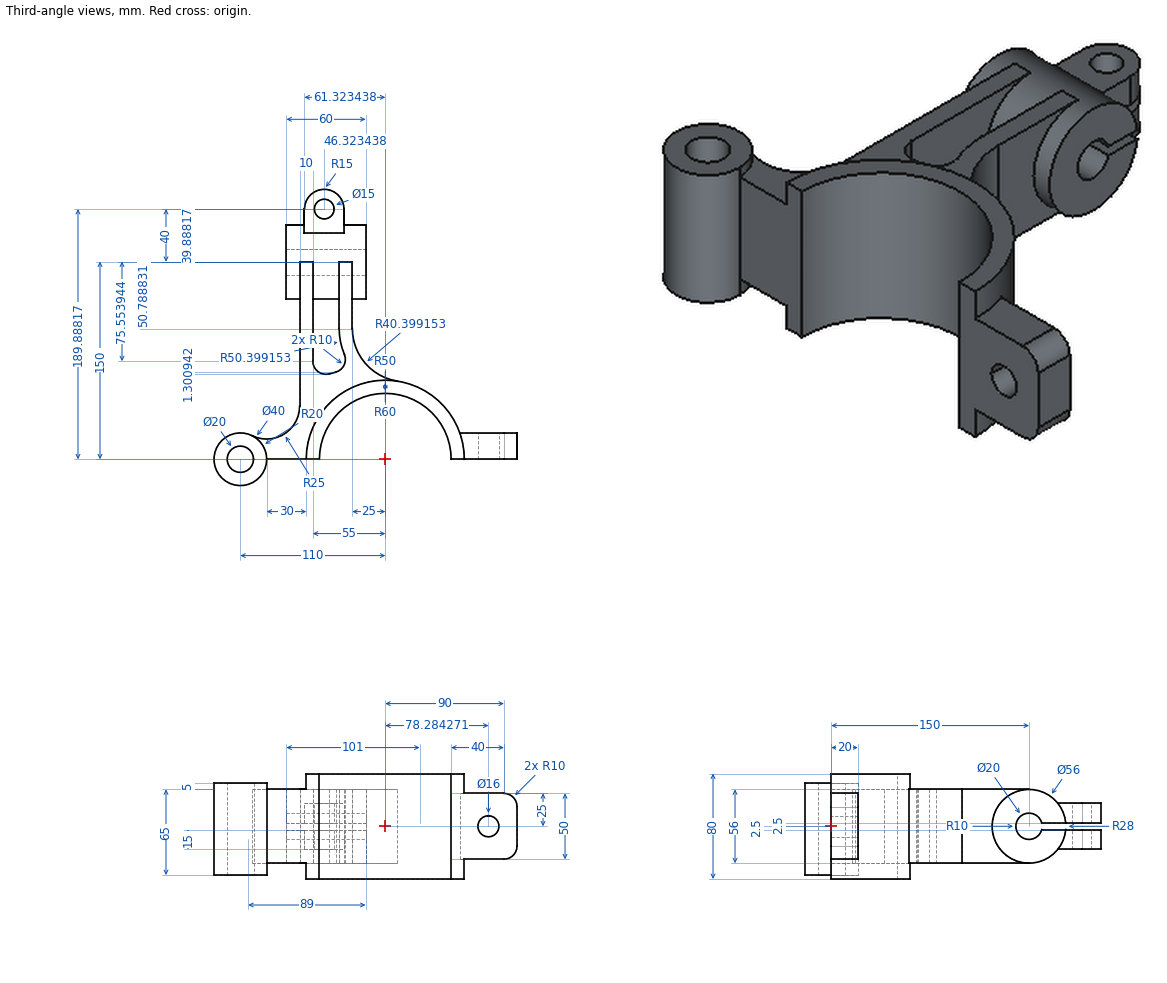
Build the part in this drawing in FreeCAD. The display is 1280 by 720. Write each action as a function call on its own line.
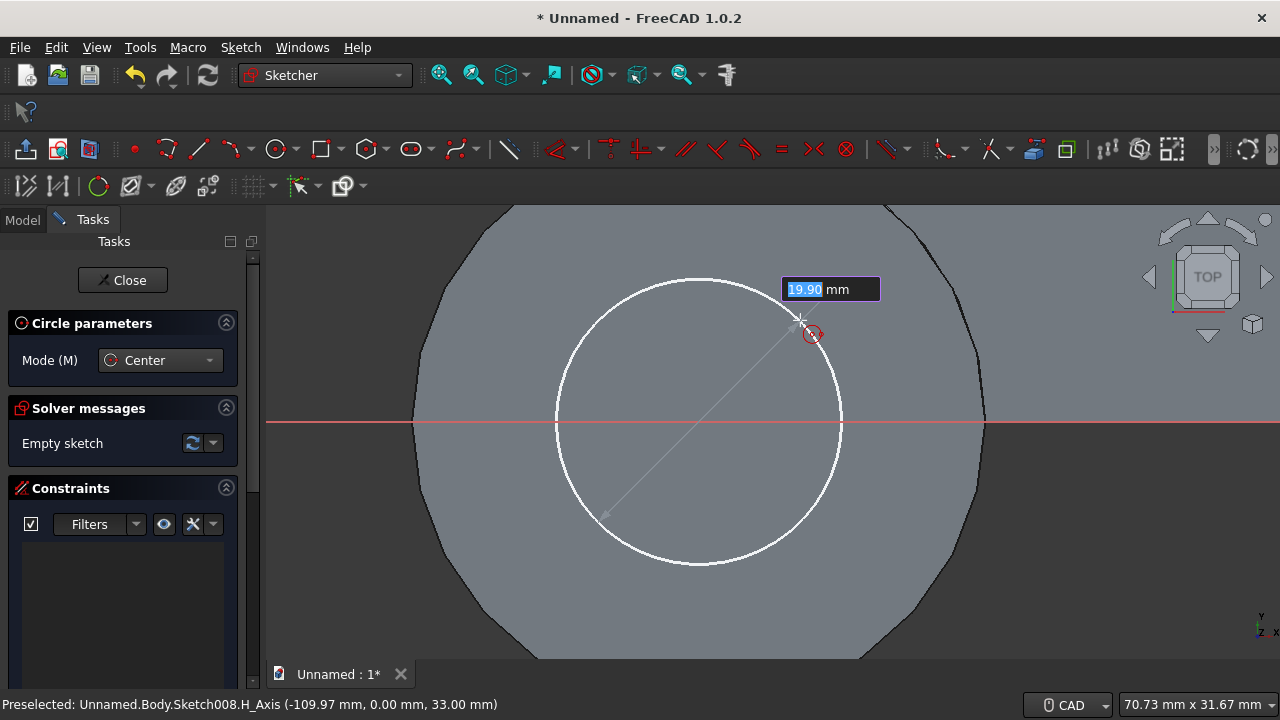
text(20)
key(Return)
key(Escape)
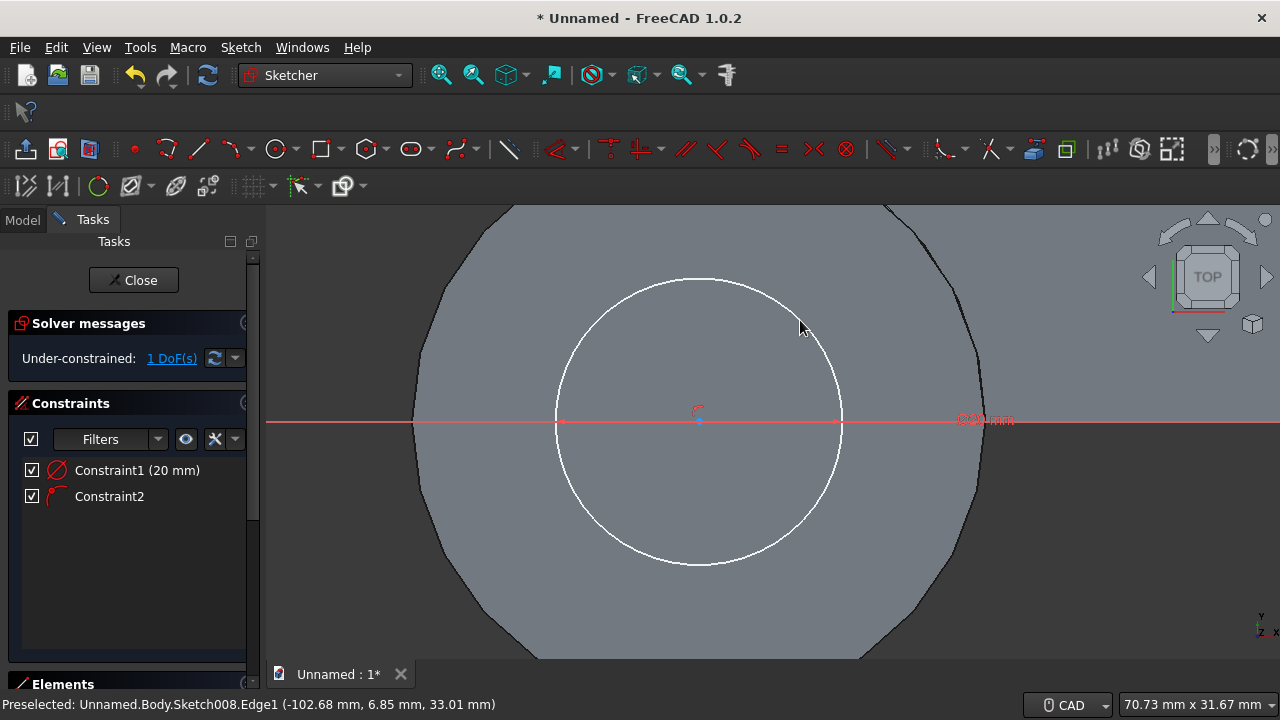
key(d)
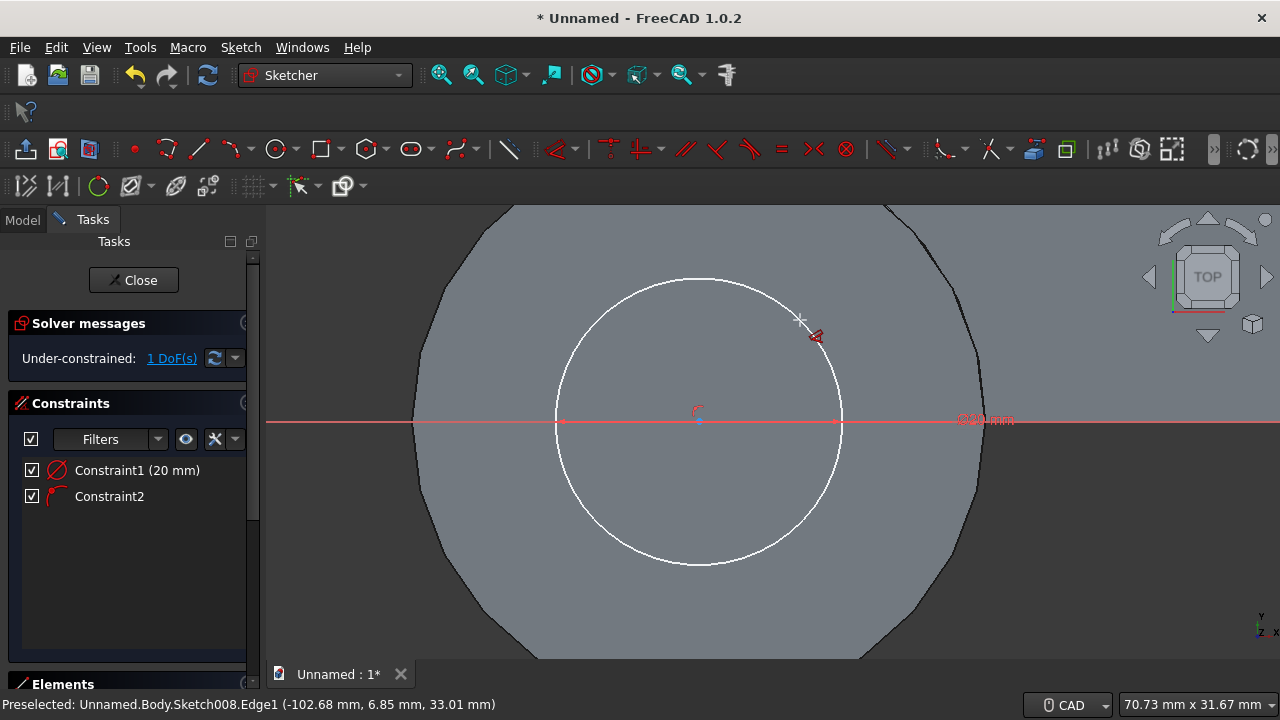
click(699, 422)
click(907, 456)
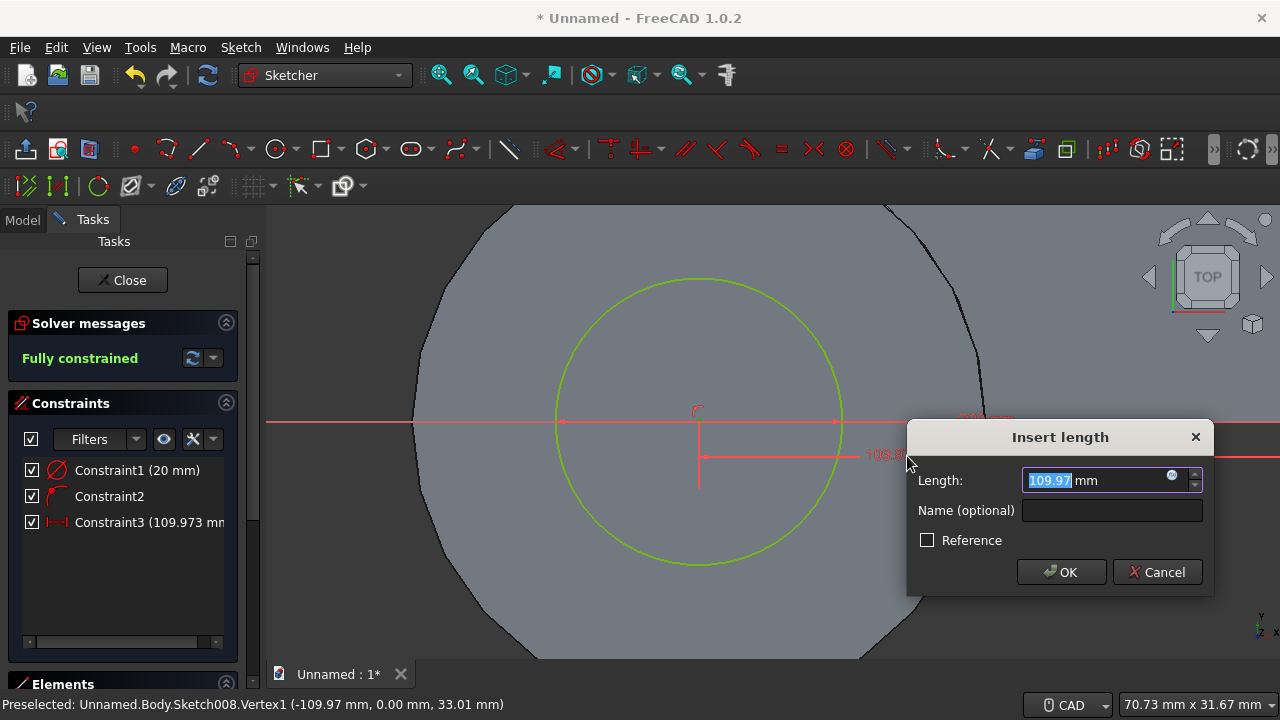
text(110)
key(Return)
key(Escape)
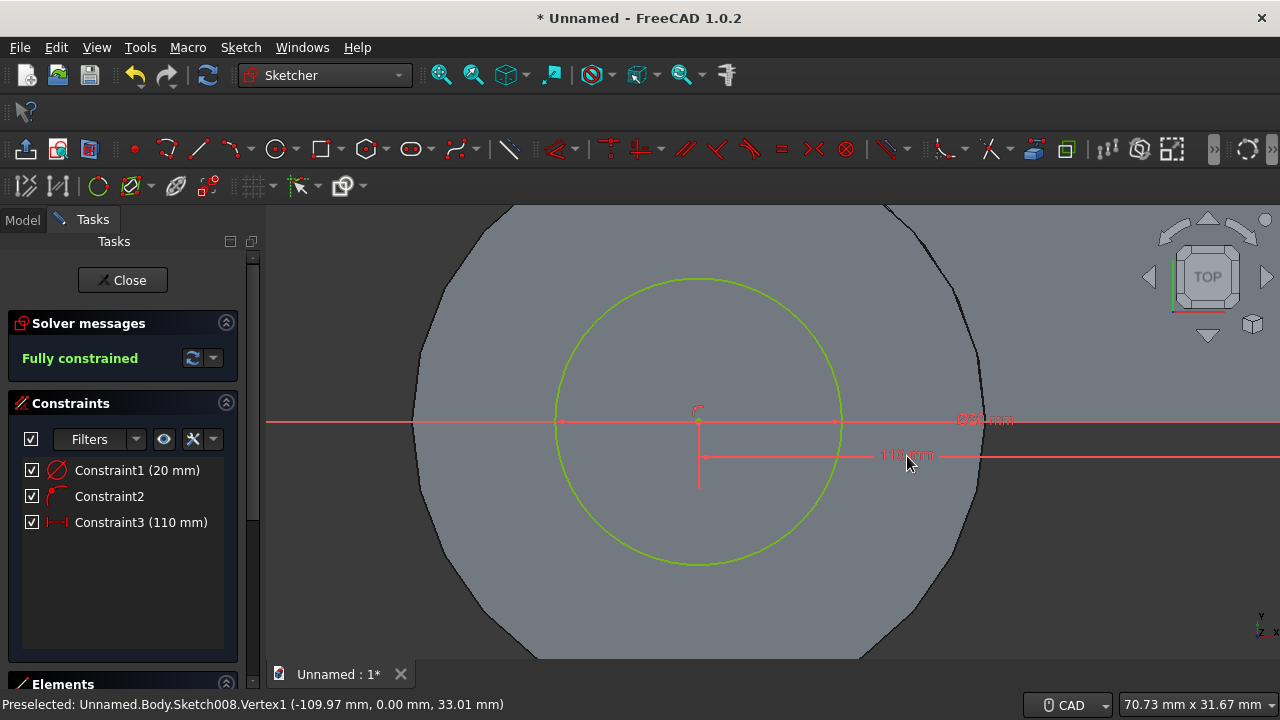
click(123, 280)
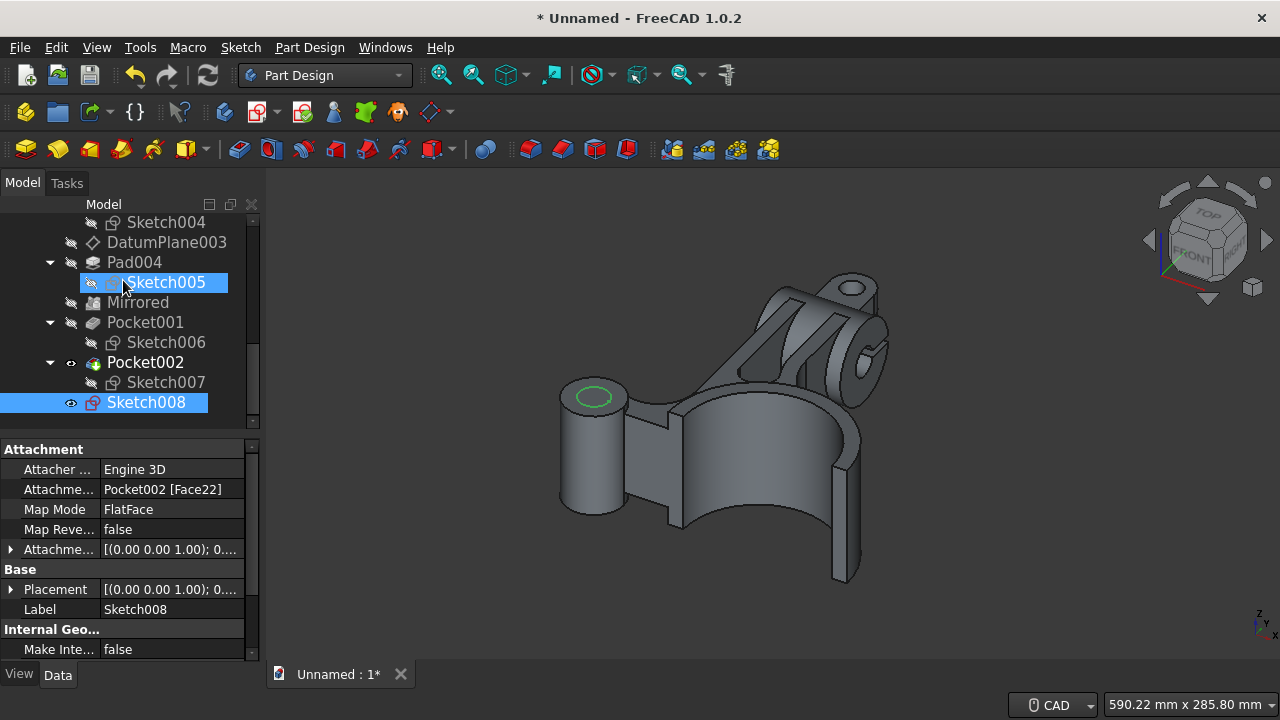
click(240, 150)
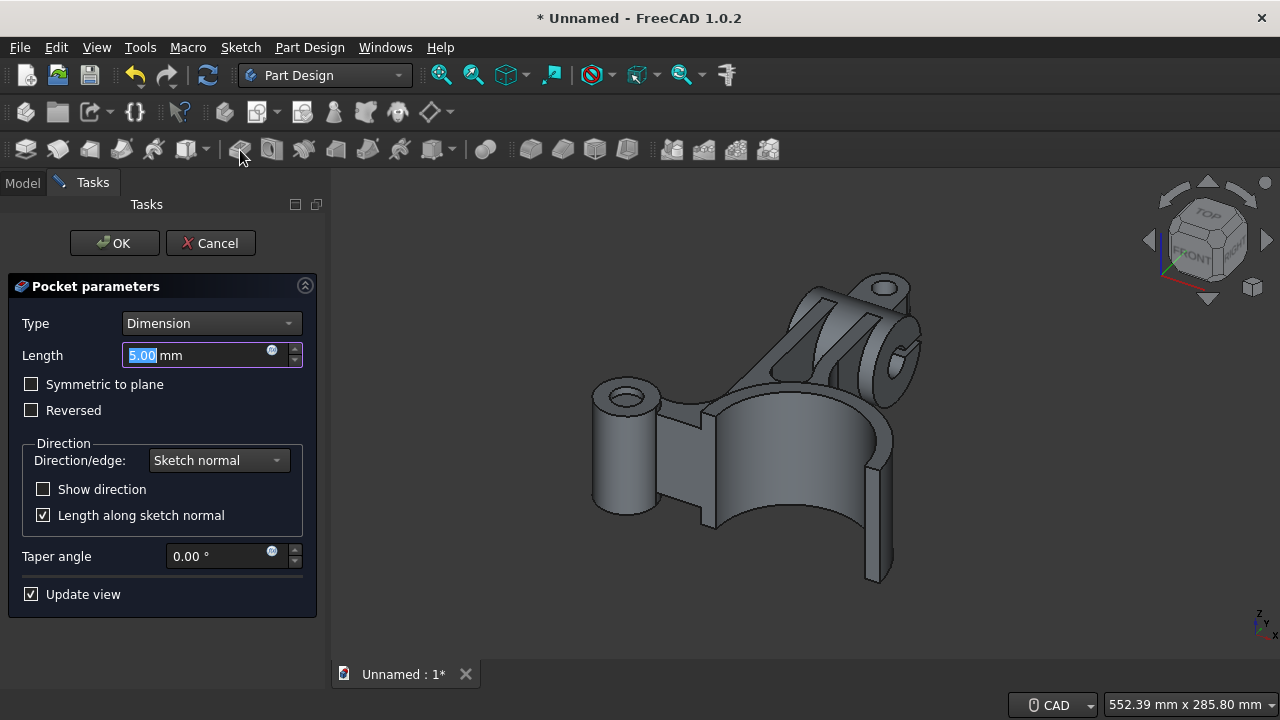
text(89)
key(Tab)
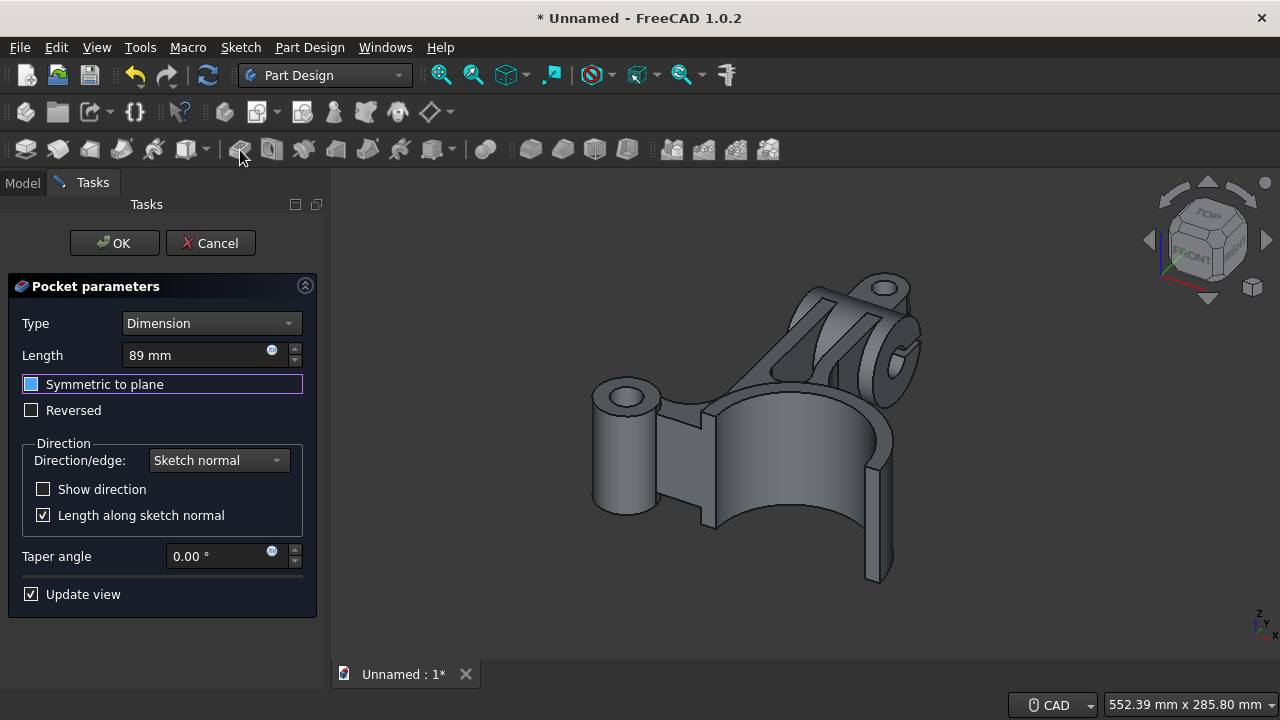
click(115, 243)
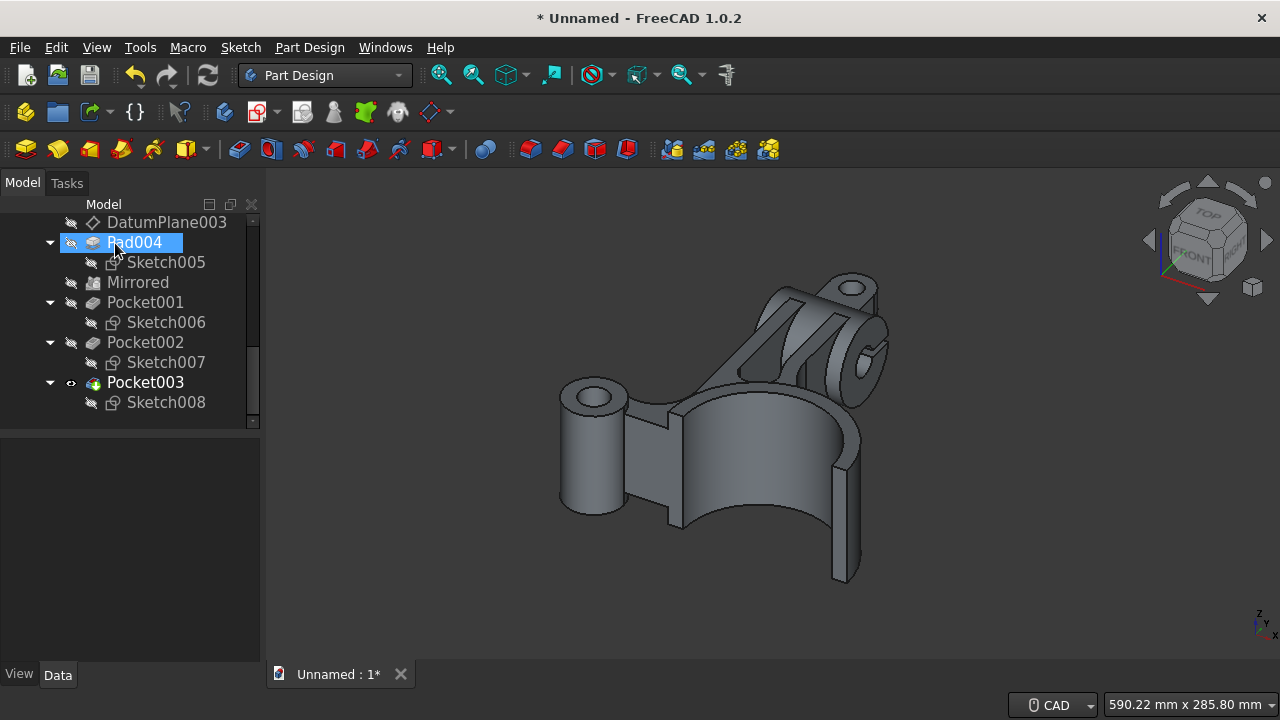
click(258, 112)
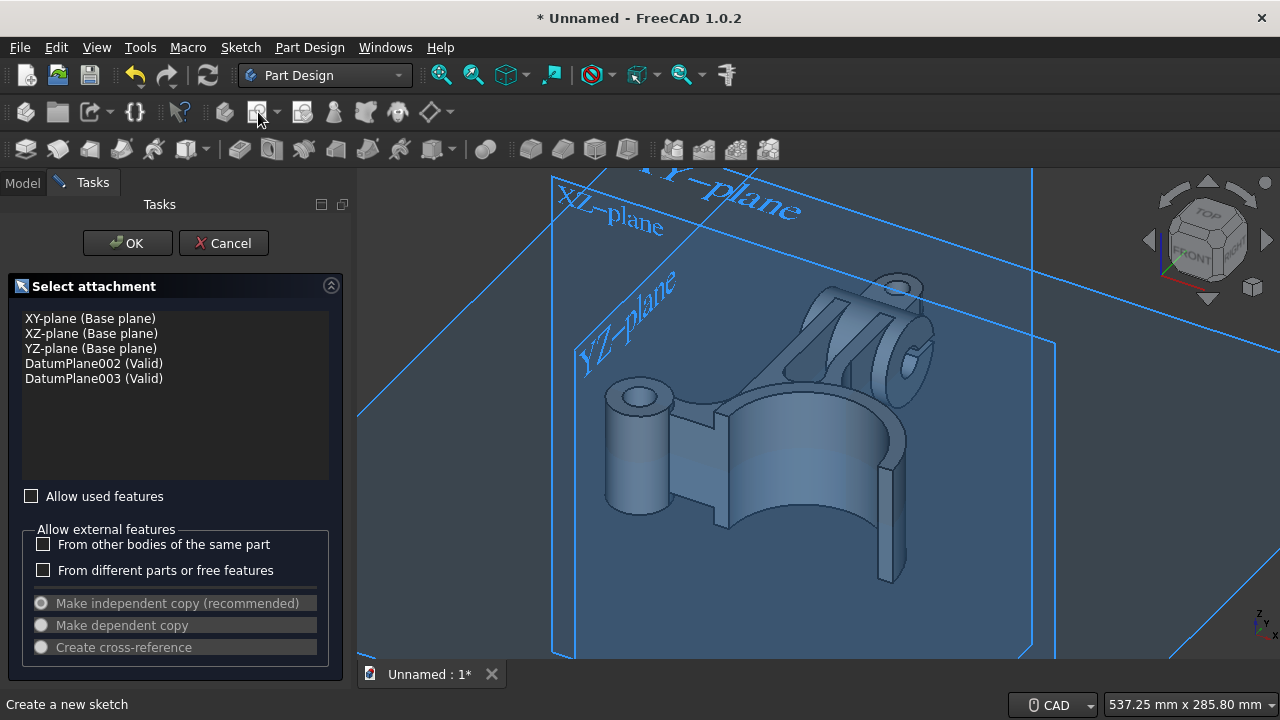
click(82, 334)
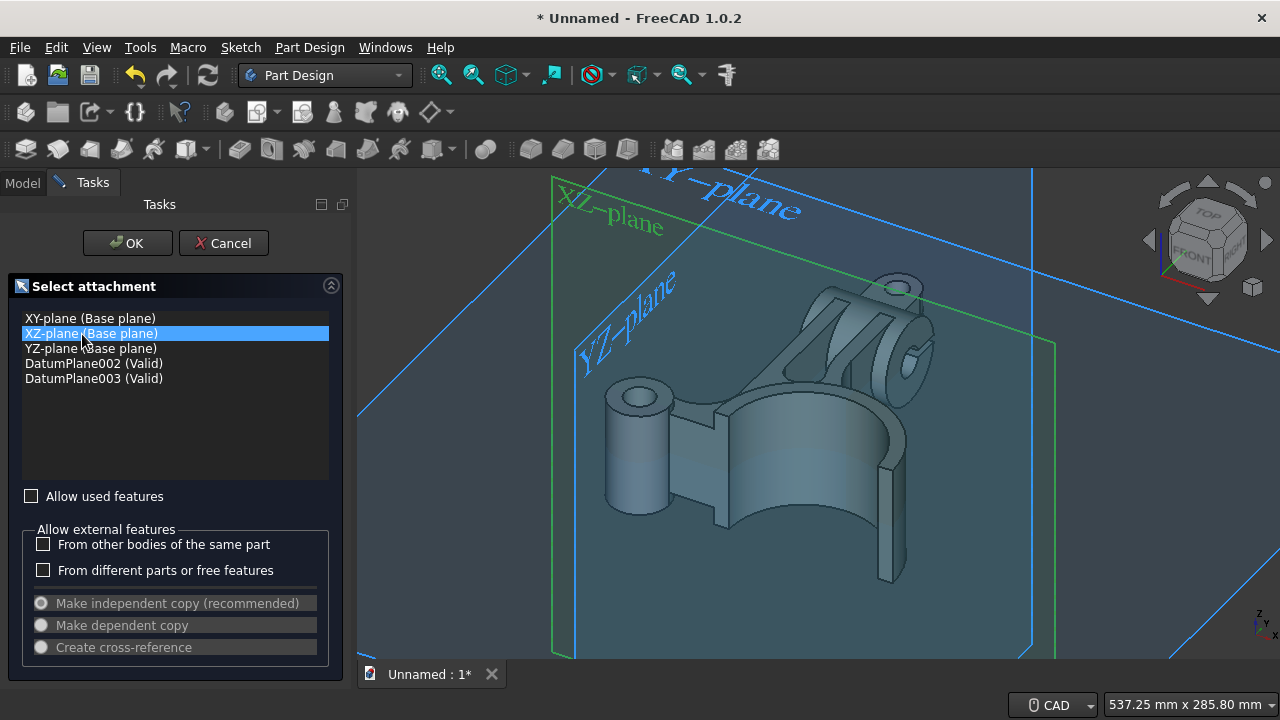
click(128, 243)